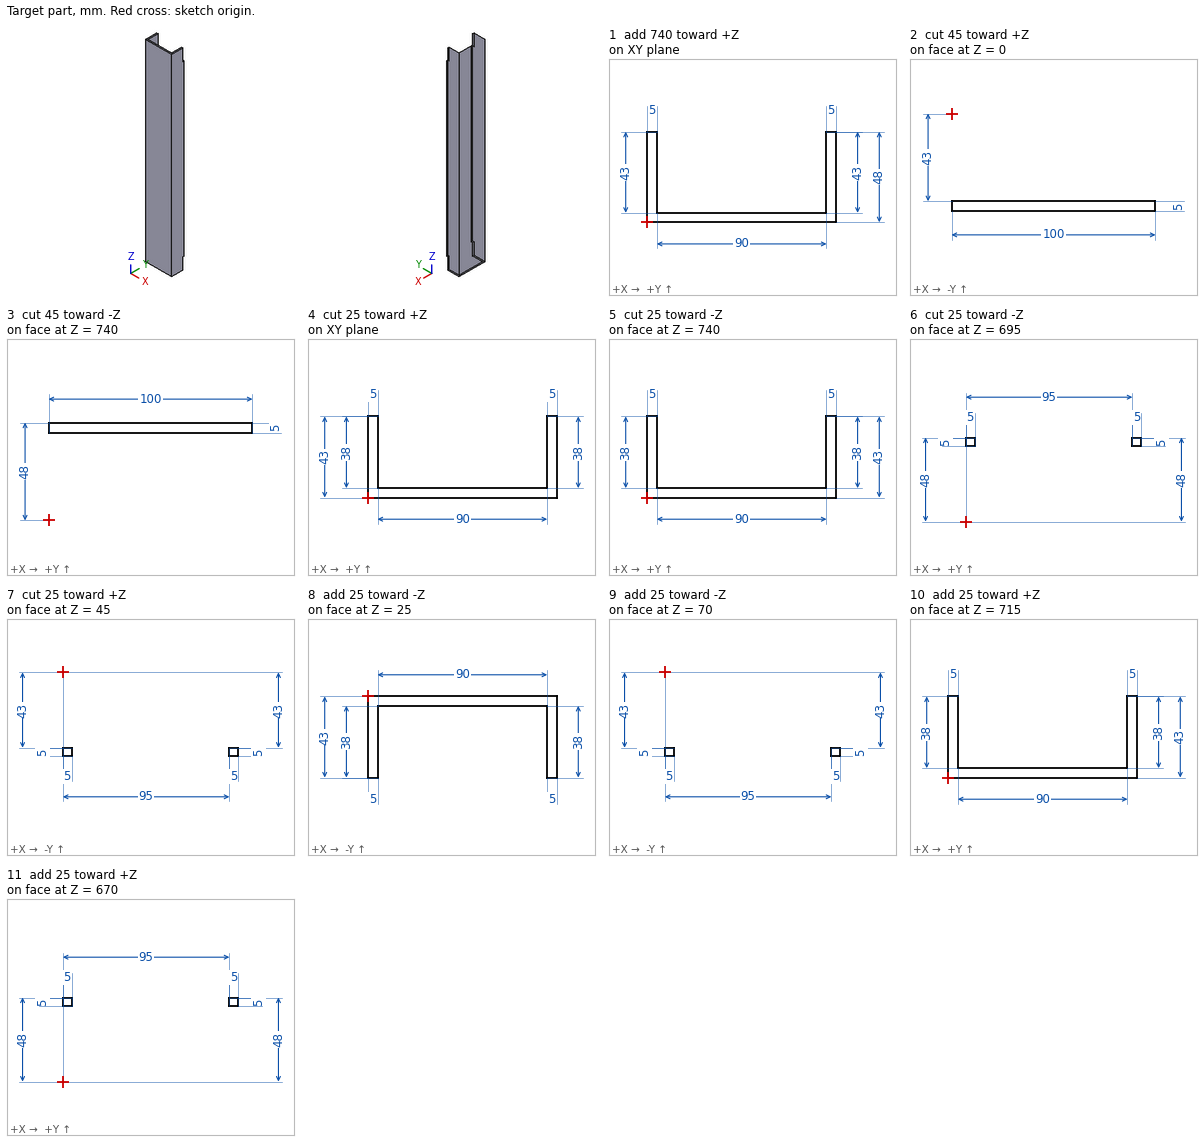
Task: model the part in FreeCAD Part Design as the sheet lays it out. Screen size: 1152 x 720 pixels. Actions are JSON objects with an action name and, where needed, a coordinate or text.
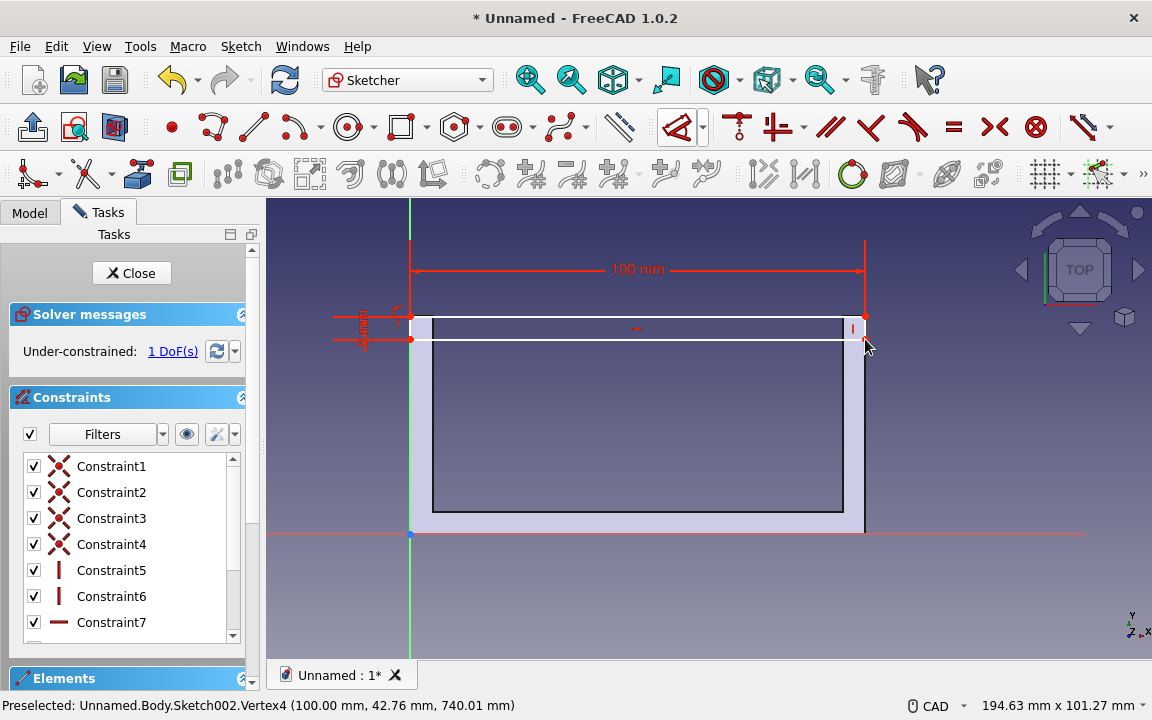
{"action": "left_click", "coordinate": [410, 317]}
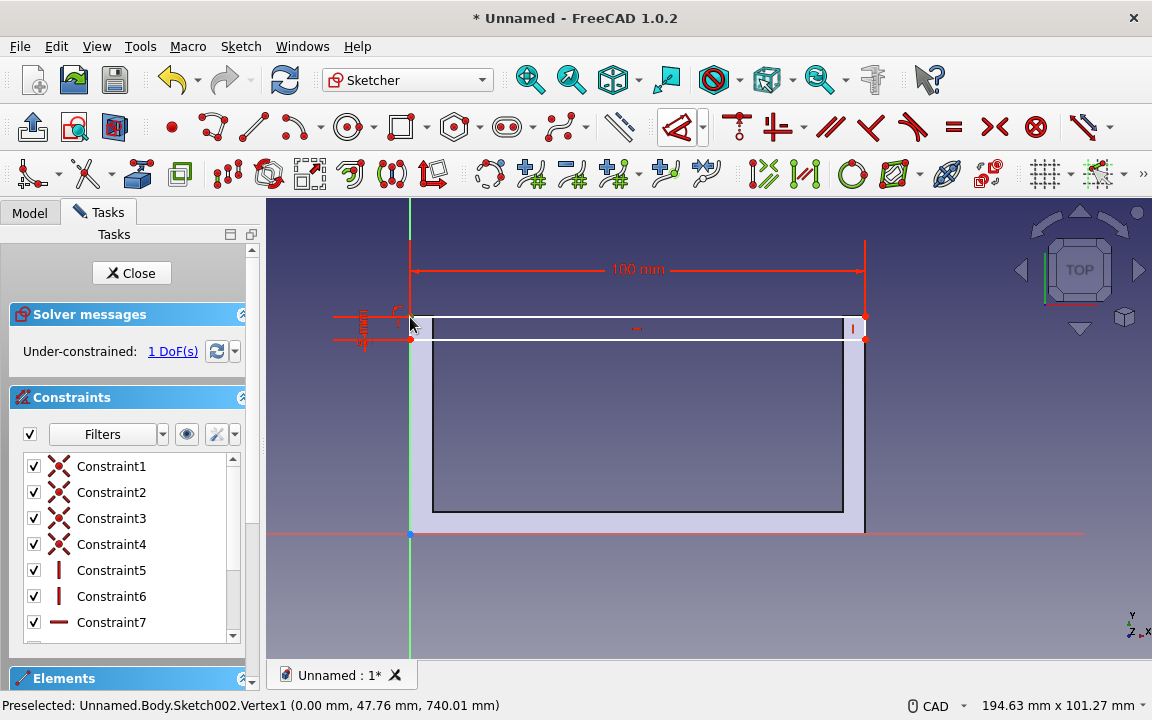
{"action": "key", "text": "i"}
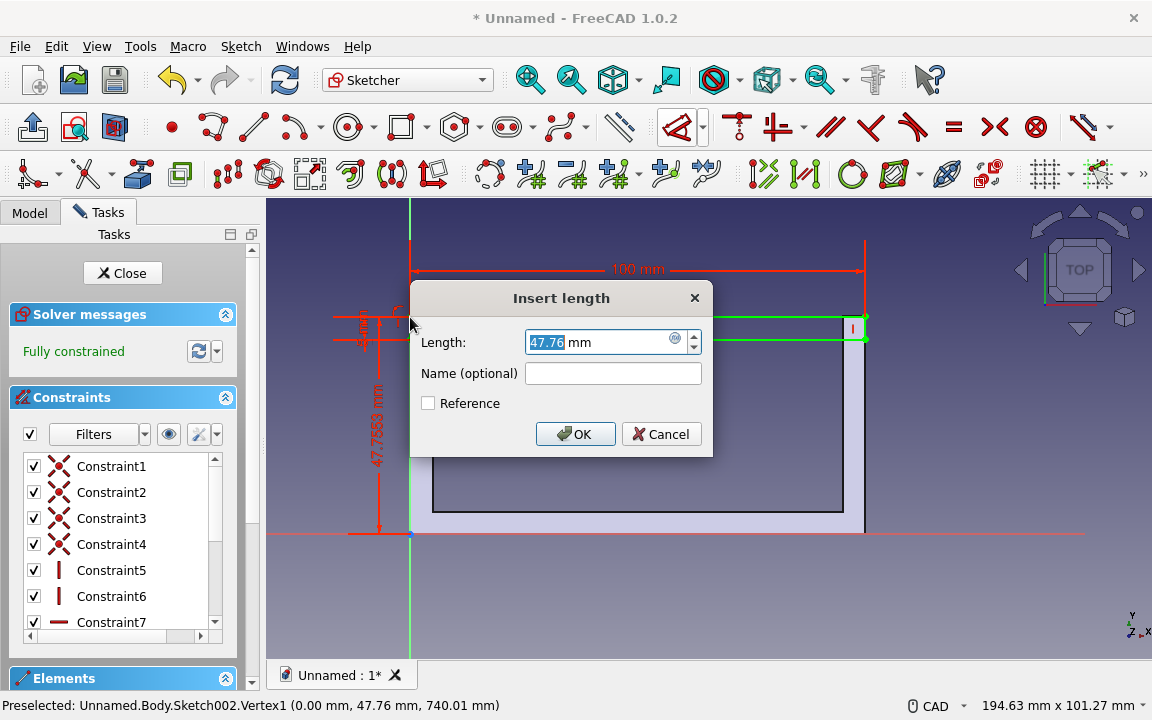
{"action": "type", "text": "48"}
{"action": "key", "text": "Return"}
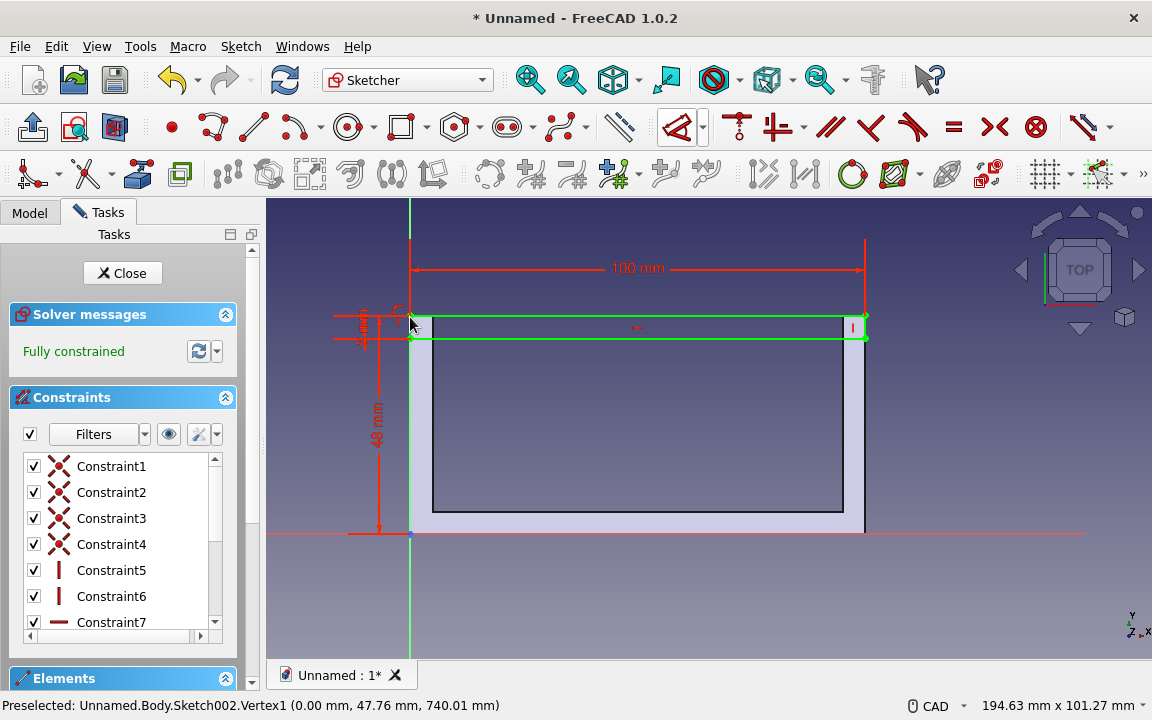
{"action": "left_click", "coordinate": [123, 273]}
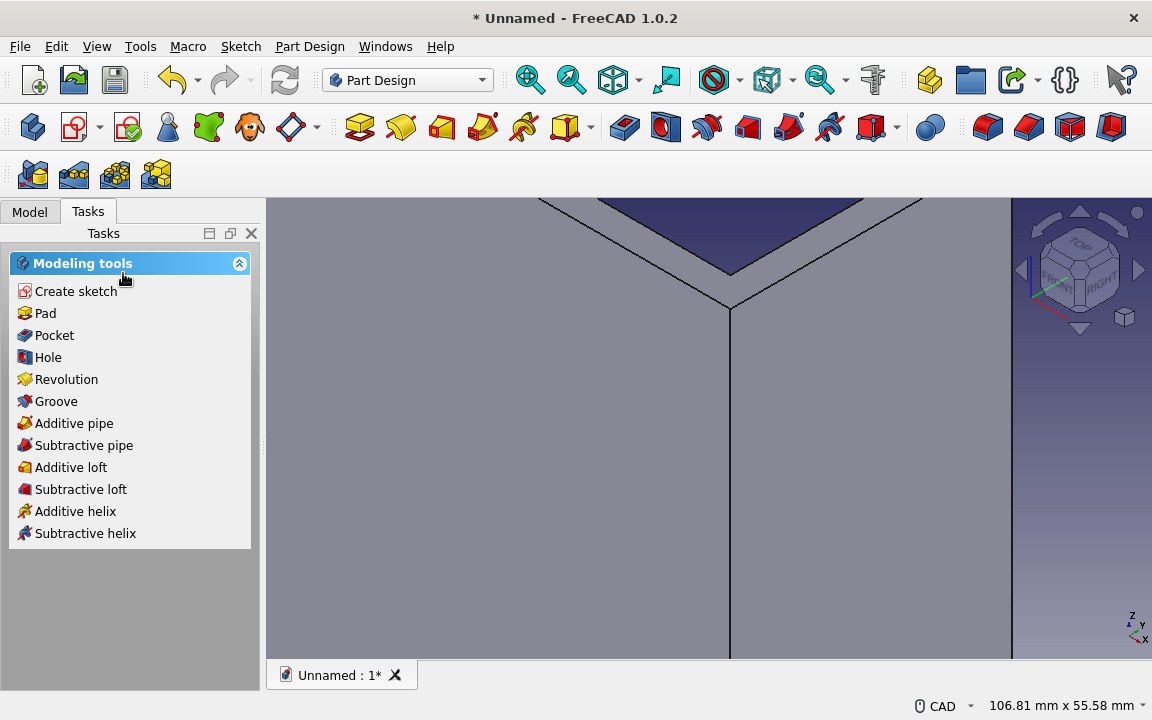
{"action": "left_click", "coordinate": [625, 128]}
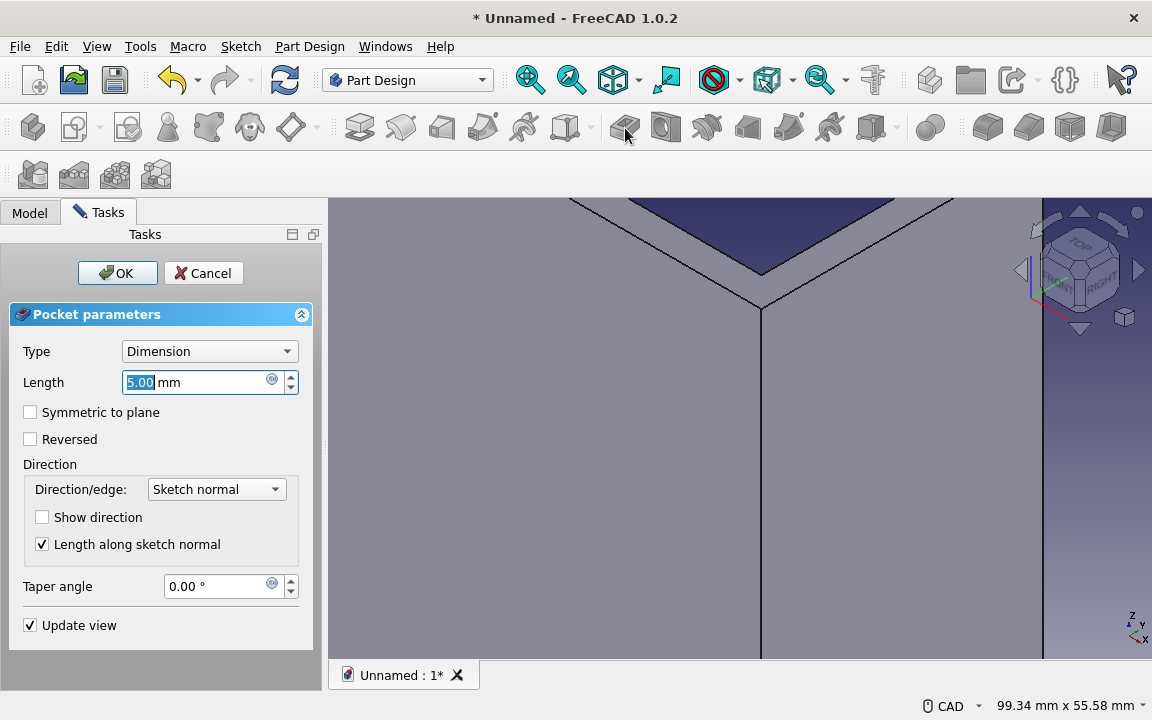
{"action": "type", "text": "45"}
{"action": "key", "text": "Tab"}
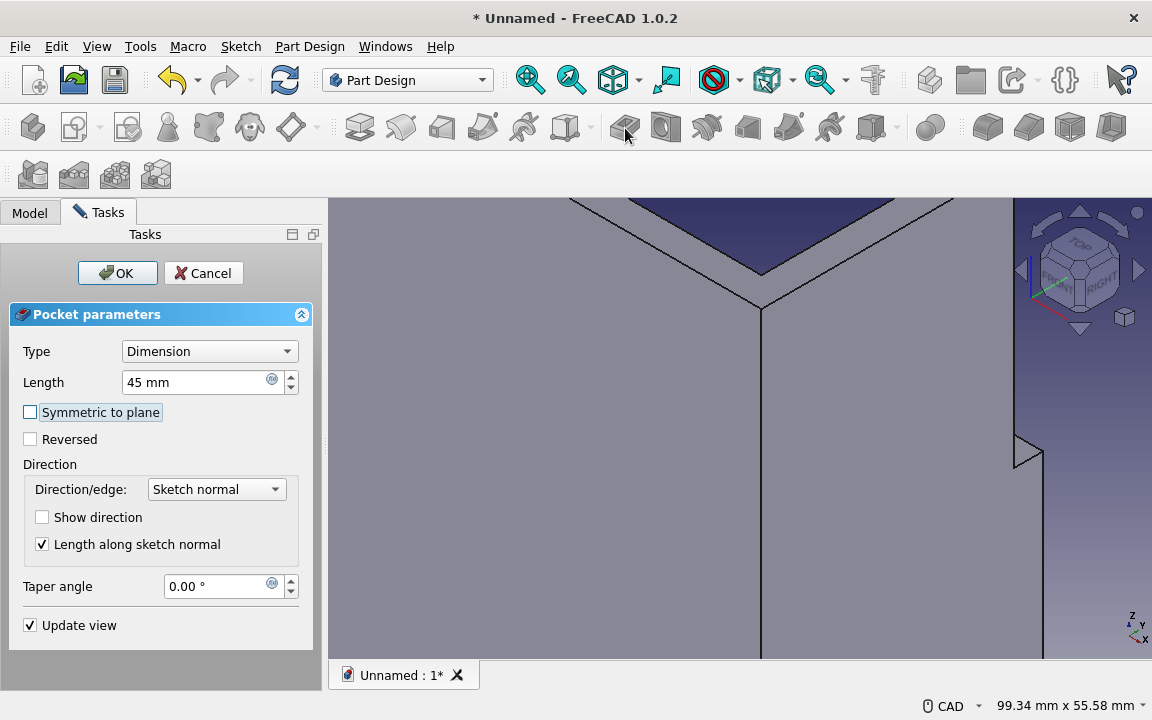
{"action": "left_click", "coordinate": [118, 273]}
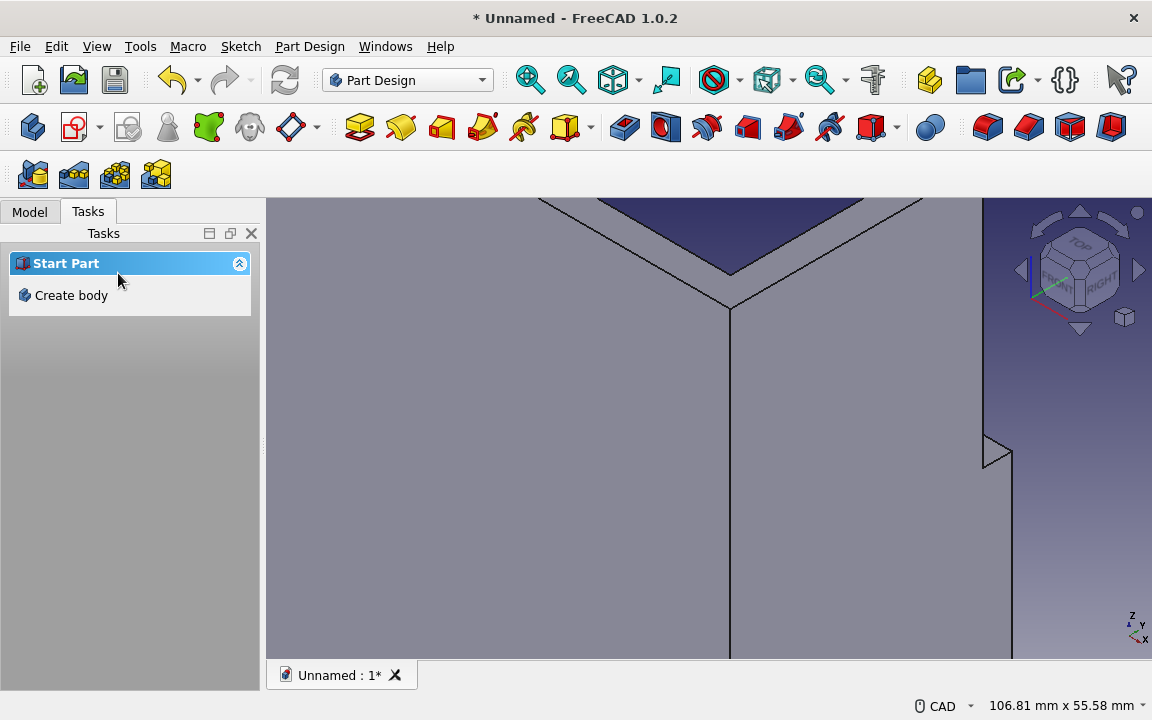
{"action": "left_click", "coordinate": [531, 80]}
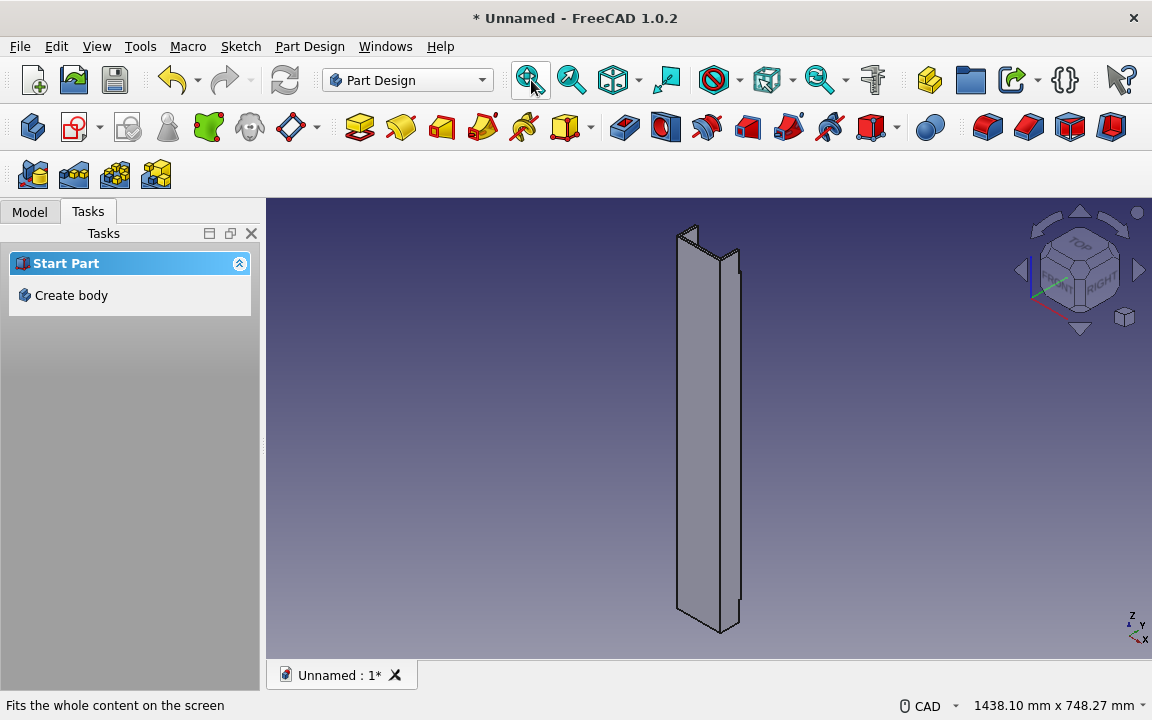
{"action": "left_click", "coordinate": [74, 128]}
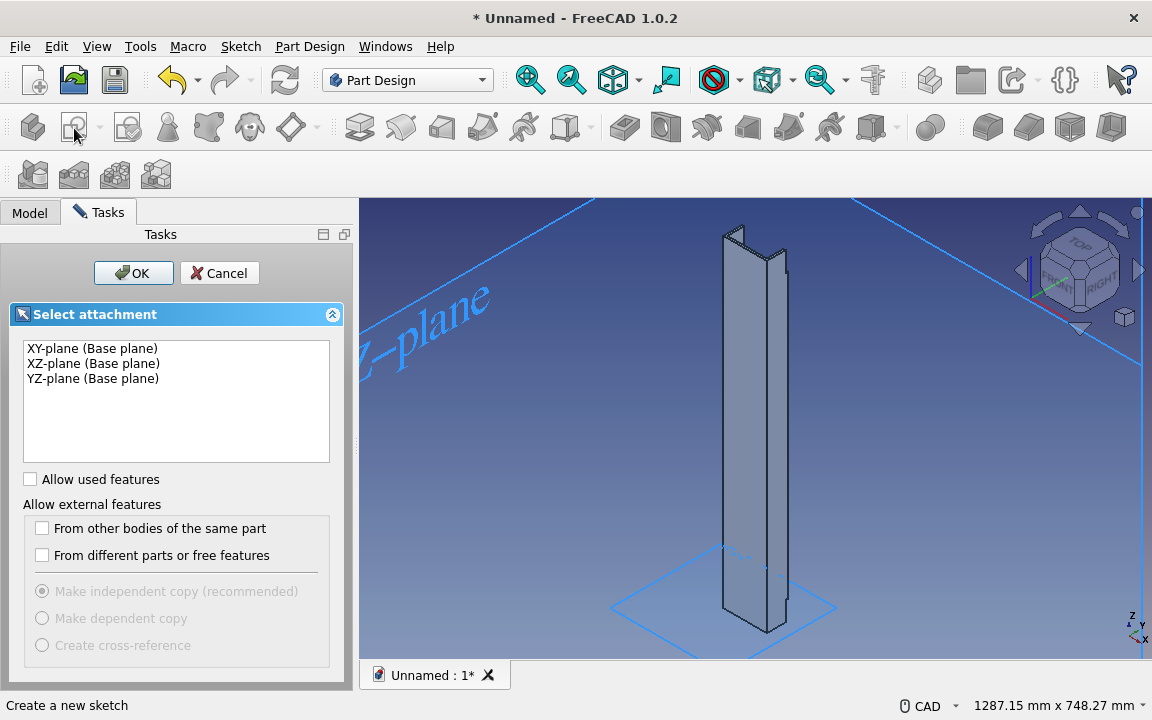
{"action": "left_click", "coordinate": [84, 348]}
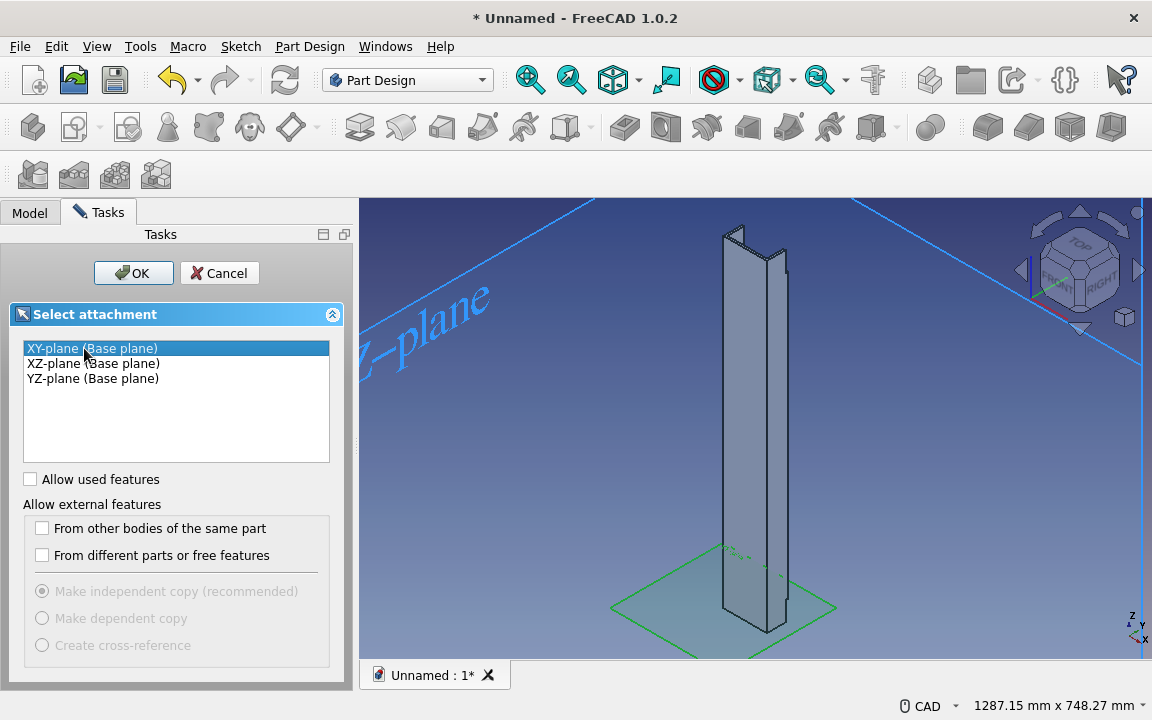
{"action": "left_click", "coordinate": [134, 273]}